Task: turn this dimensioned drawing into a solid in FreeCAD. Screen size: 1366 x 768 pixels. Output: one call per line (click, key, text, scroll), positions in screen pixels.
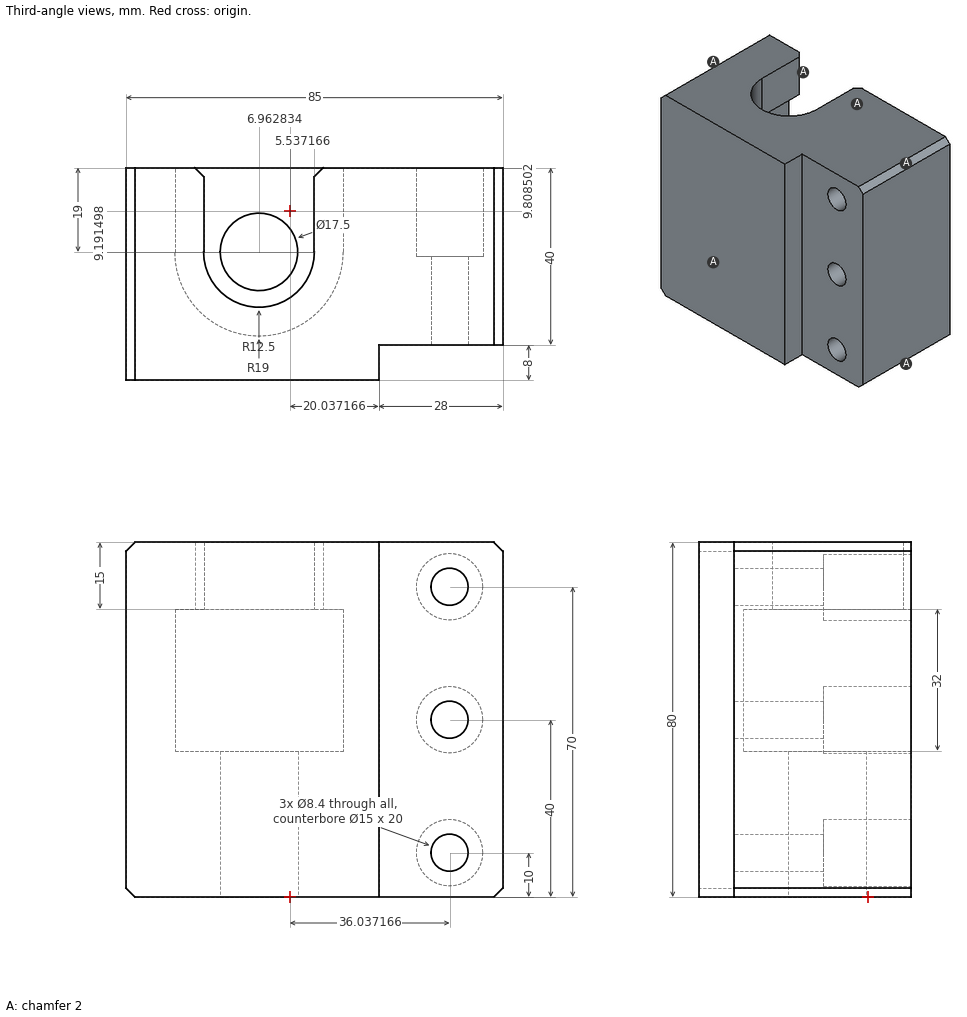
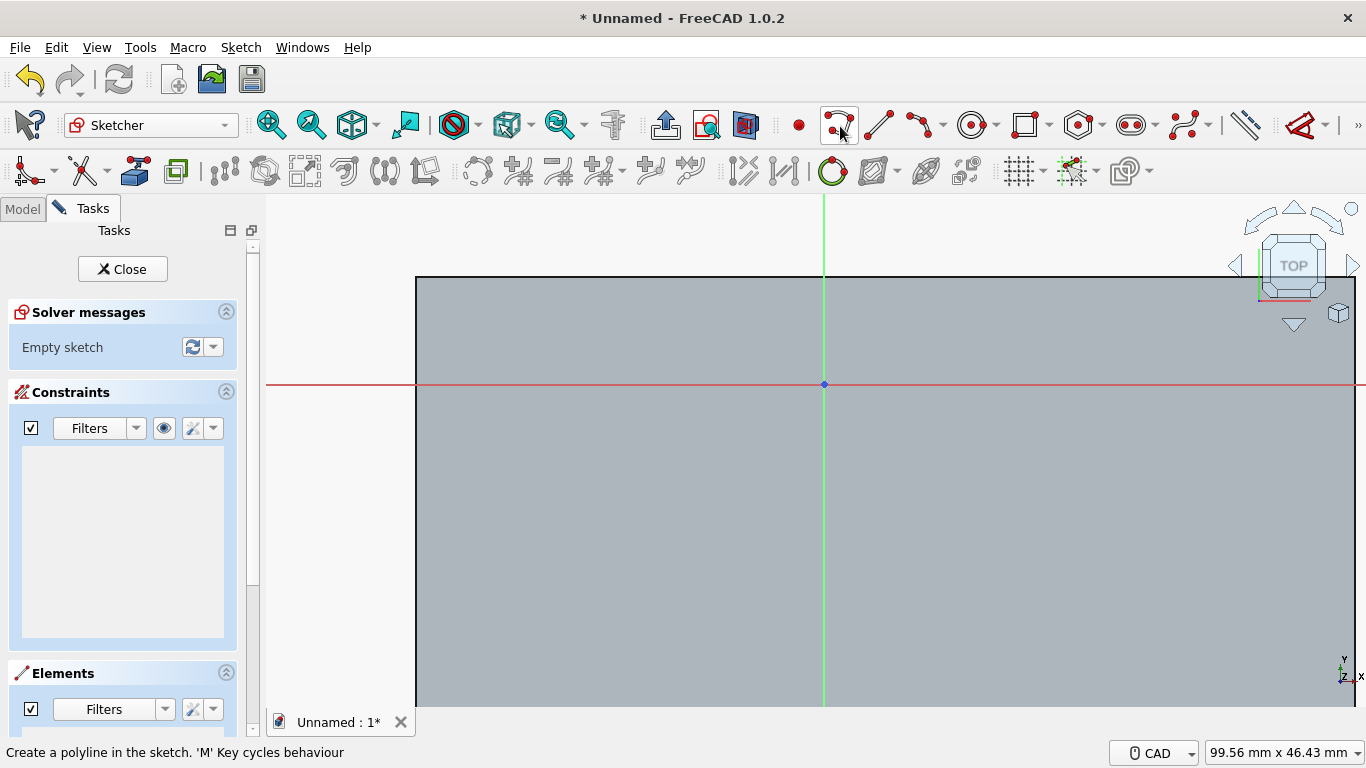
click(886, 487)
click(886, 277)
click(609, 277)
click(609, 487)
right_click(609, 487)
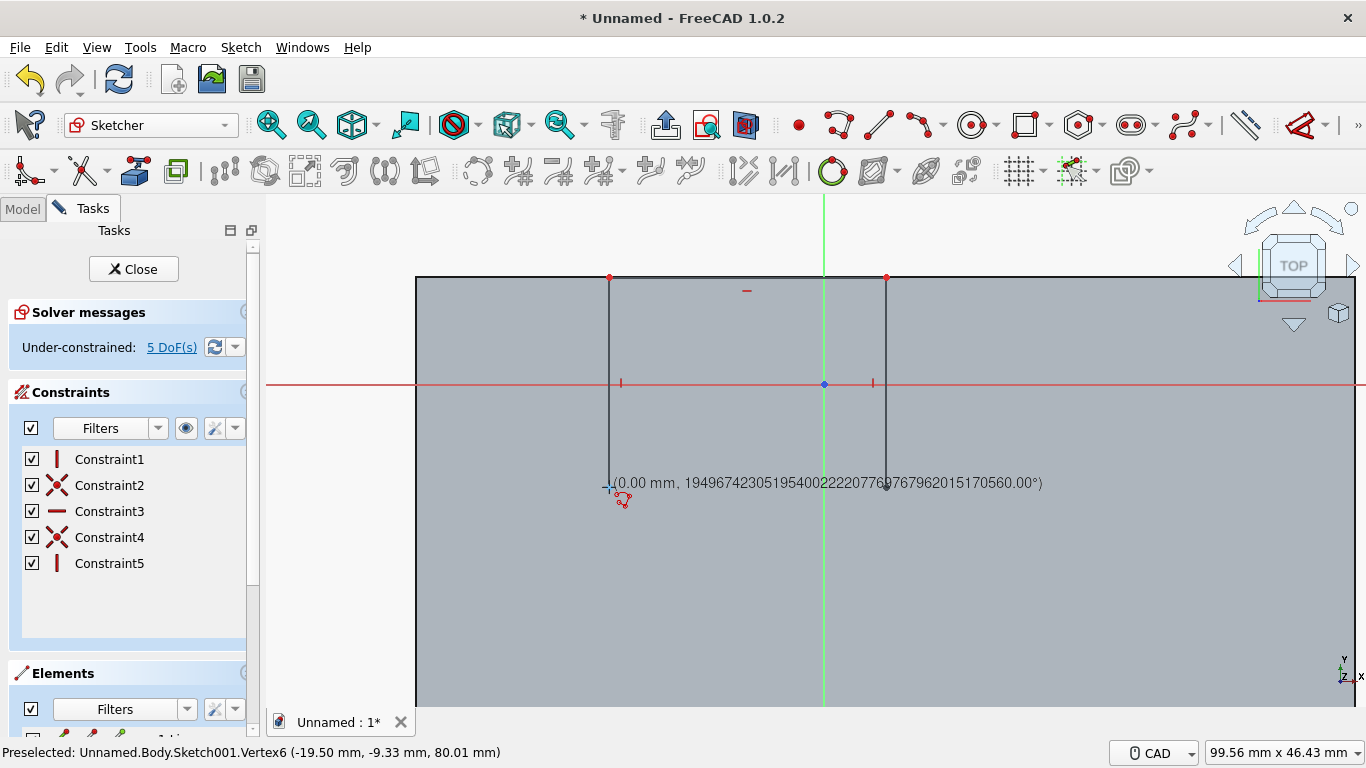
click(920, 126)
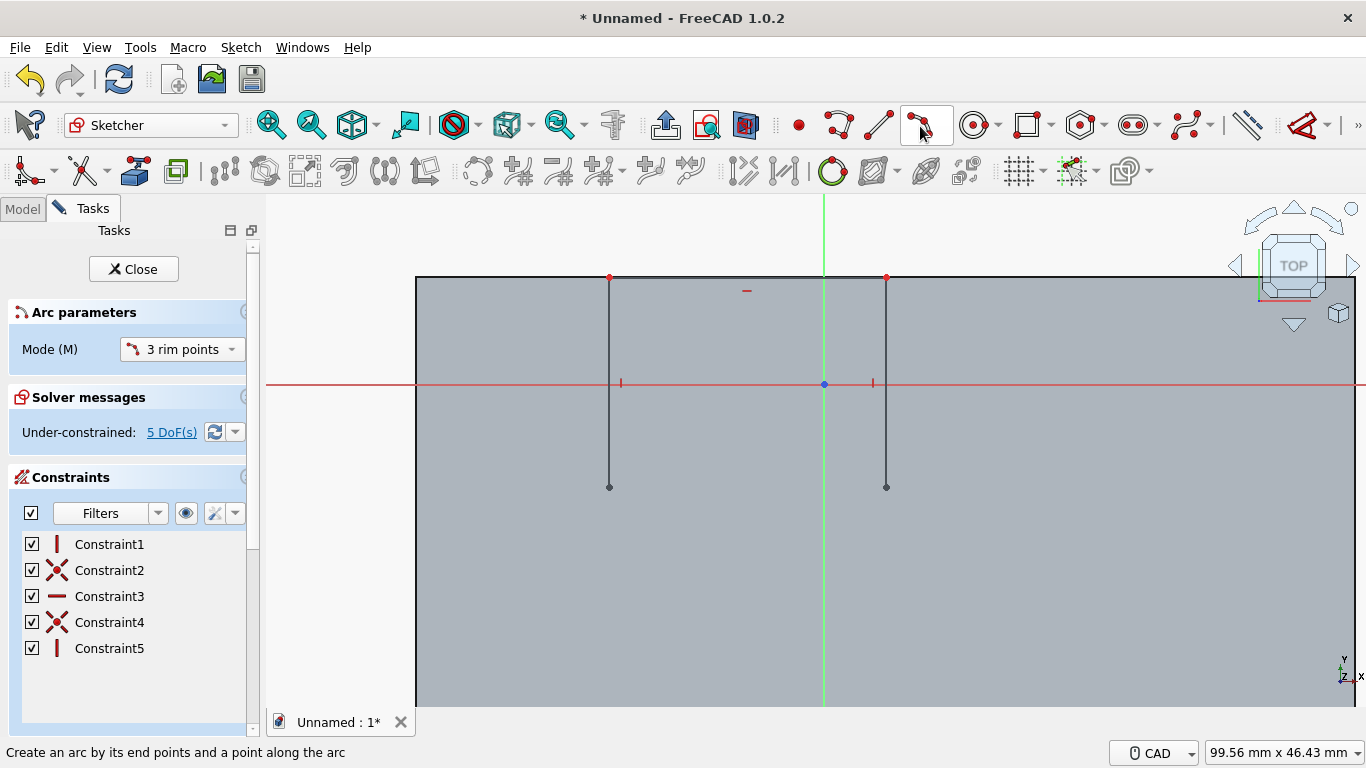
click(609, 488)
click(886, 488)
click(748, 625)
key(Escape)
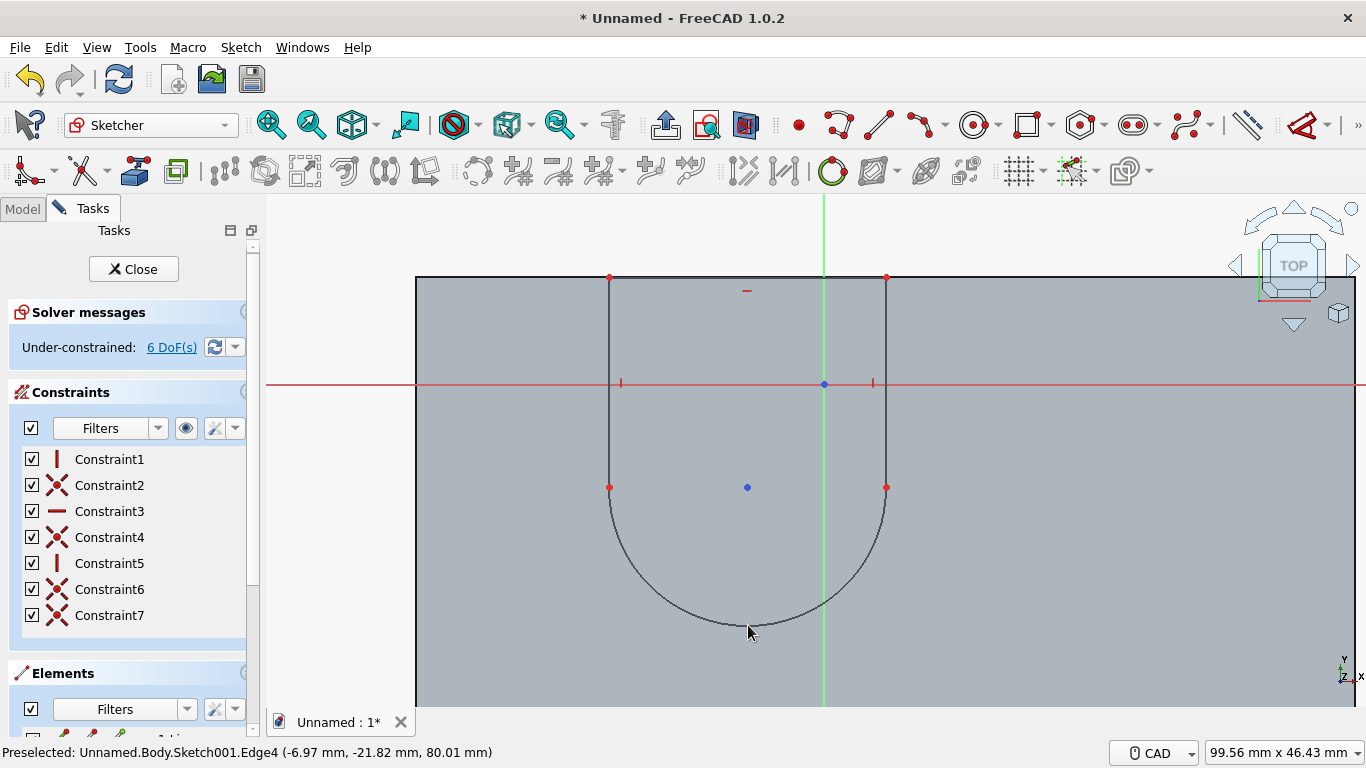
click(886, 425)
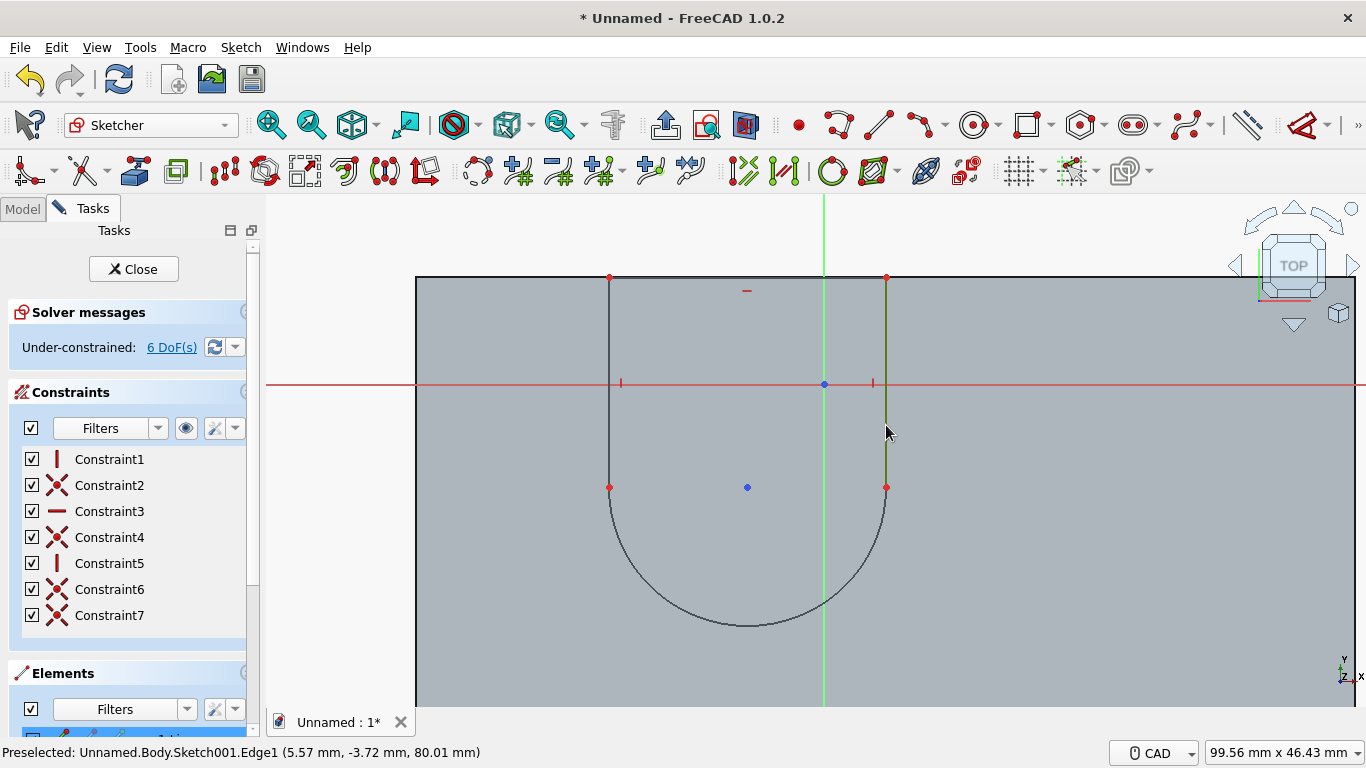
click(666, 600)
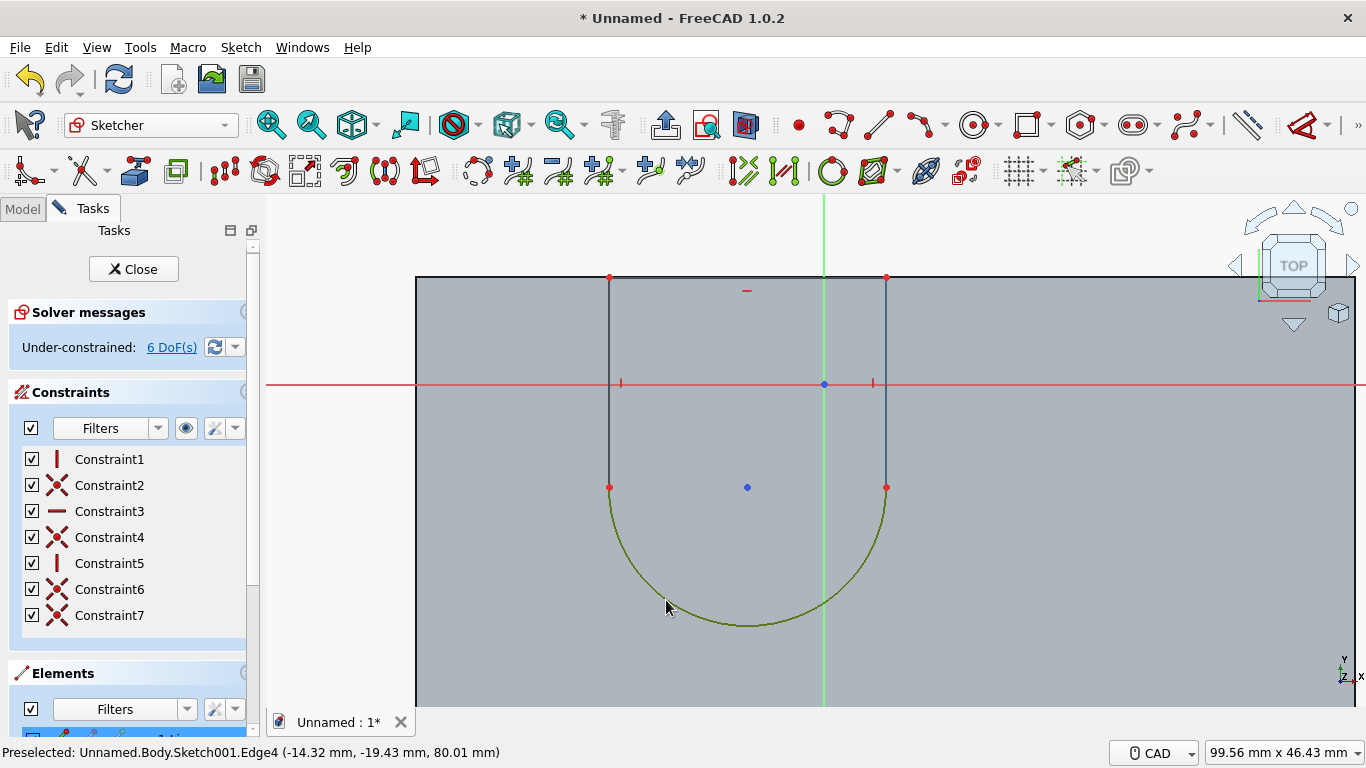
key(t)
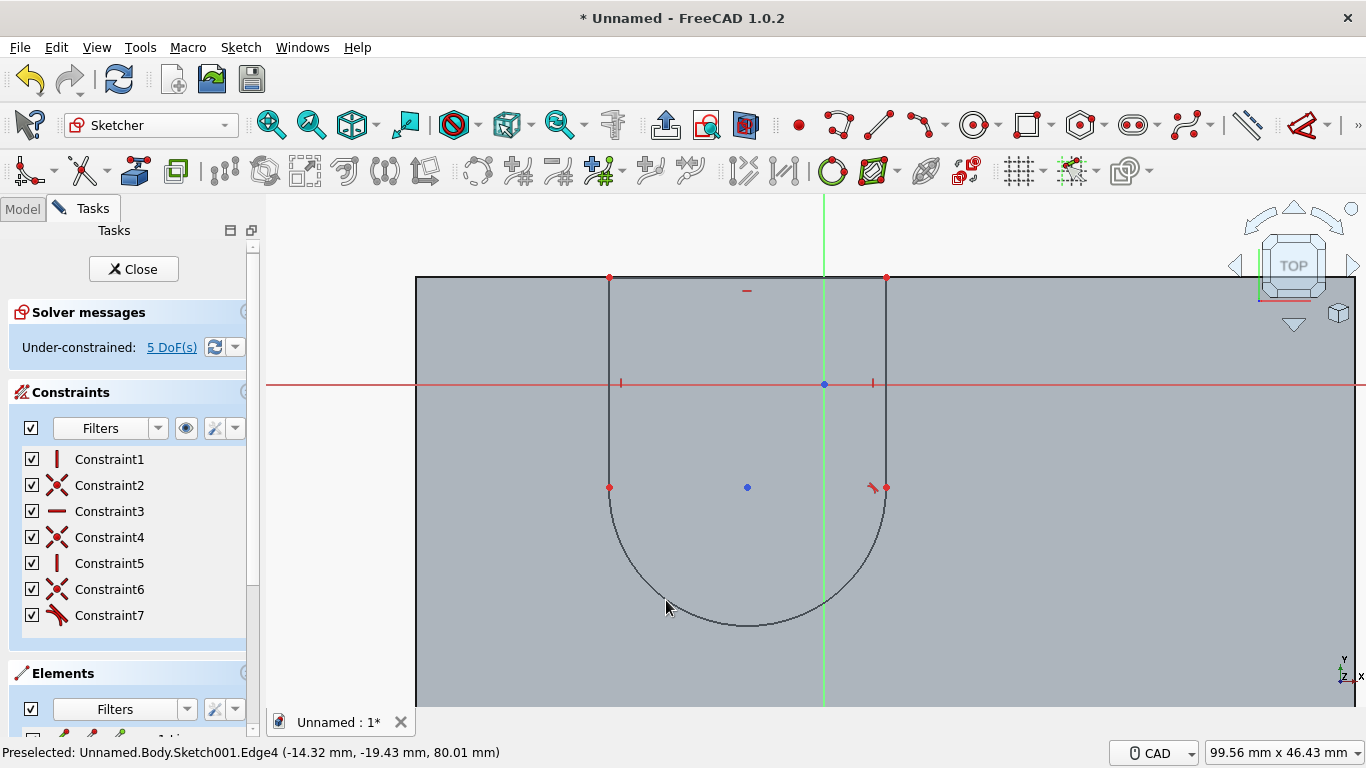
click(609, 341)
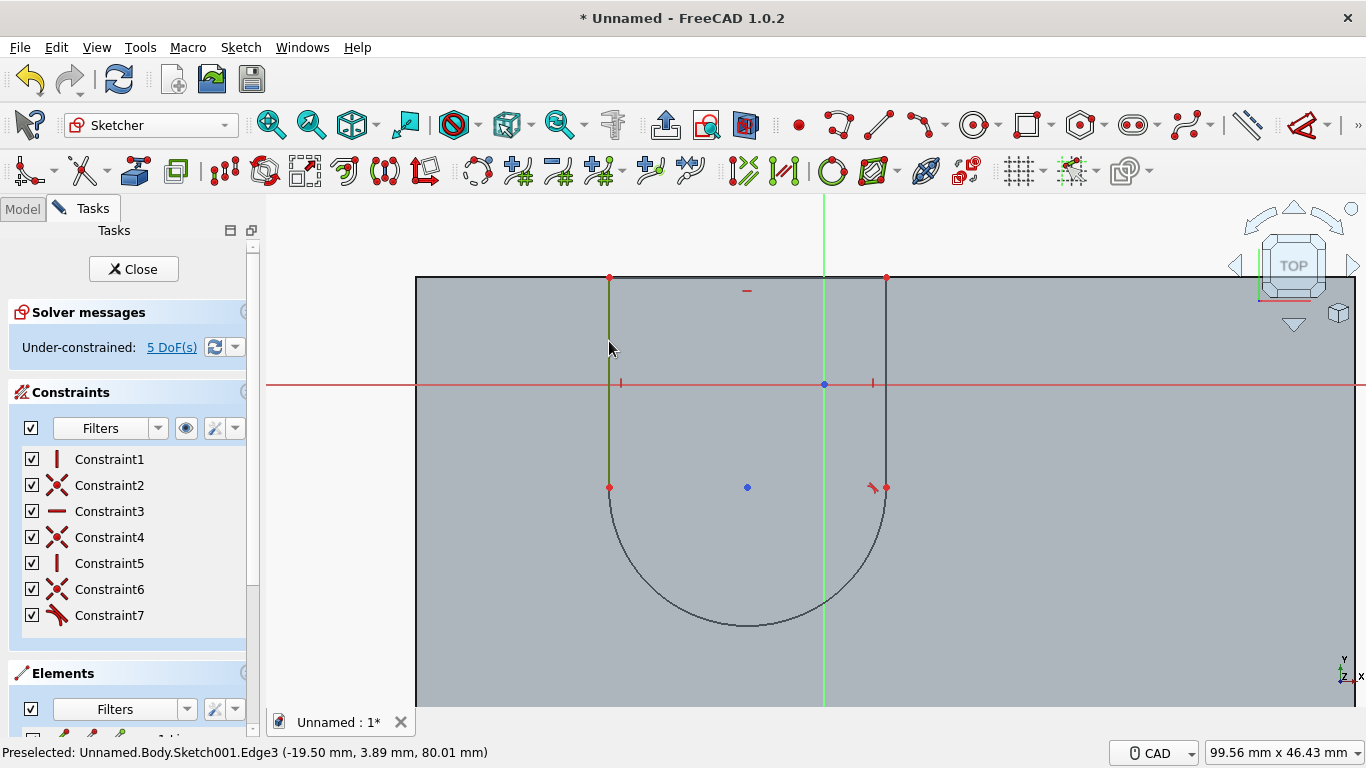
click(666, 600)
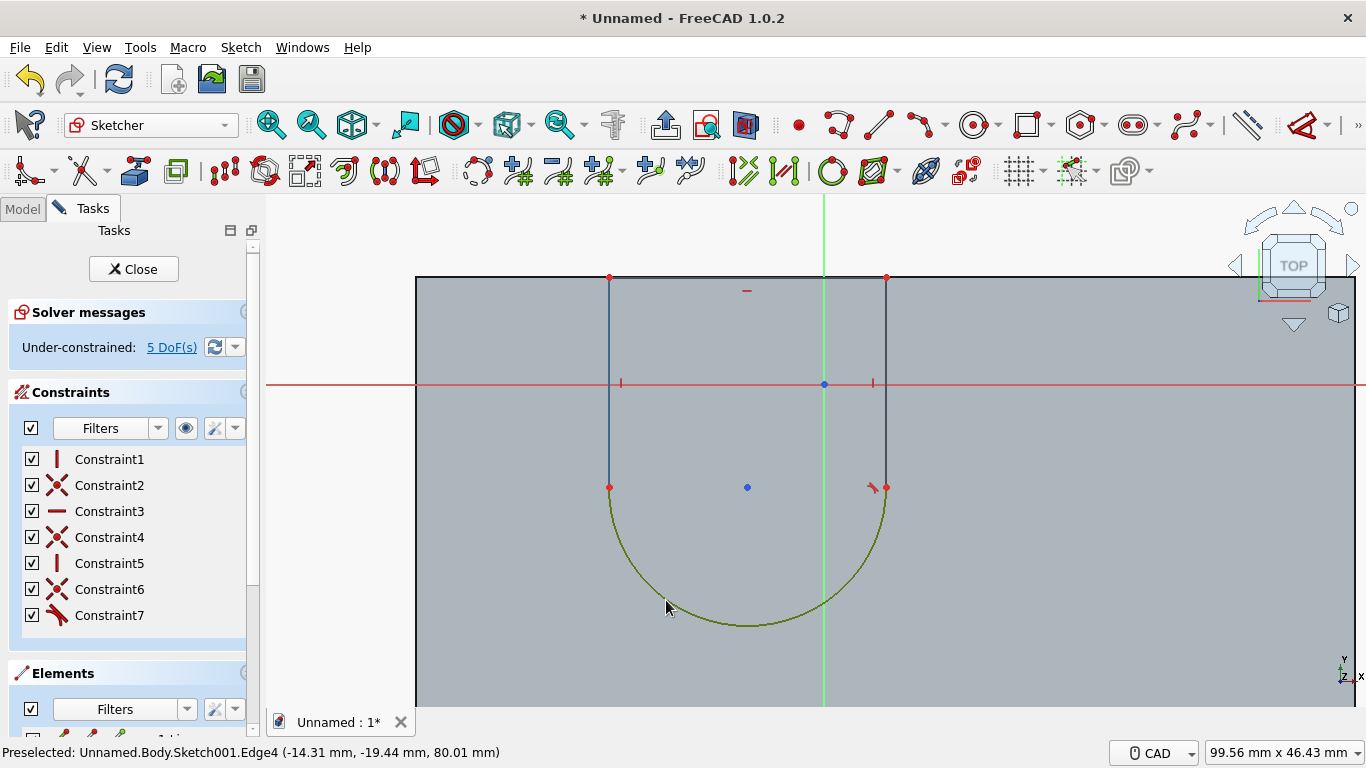
key(t)